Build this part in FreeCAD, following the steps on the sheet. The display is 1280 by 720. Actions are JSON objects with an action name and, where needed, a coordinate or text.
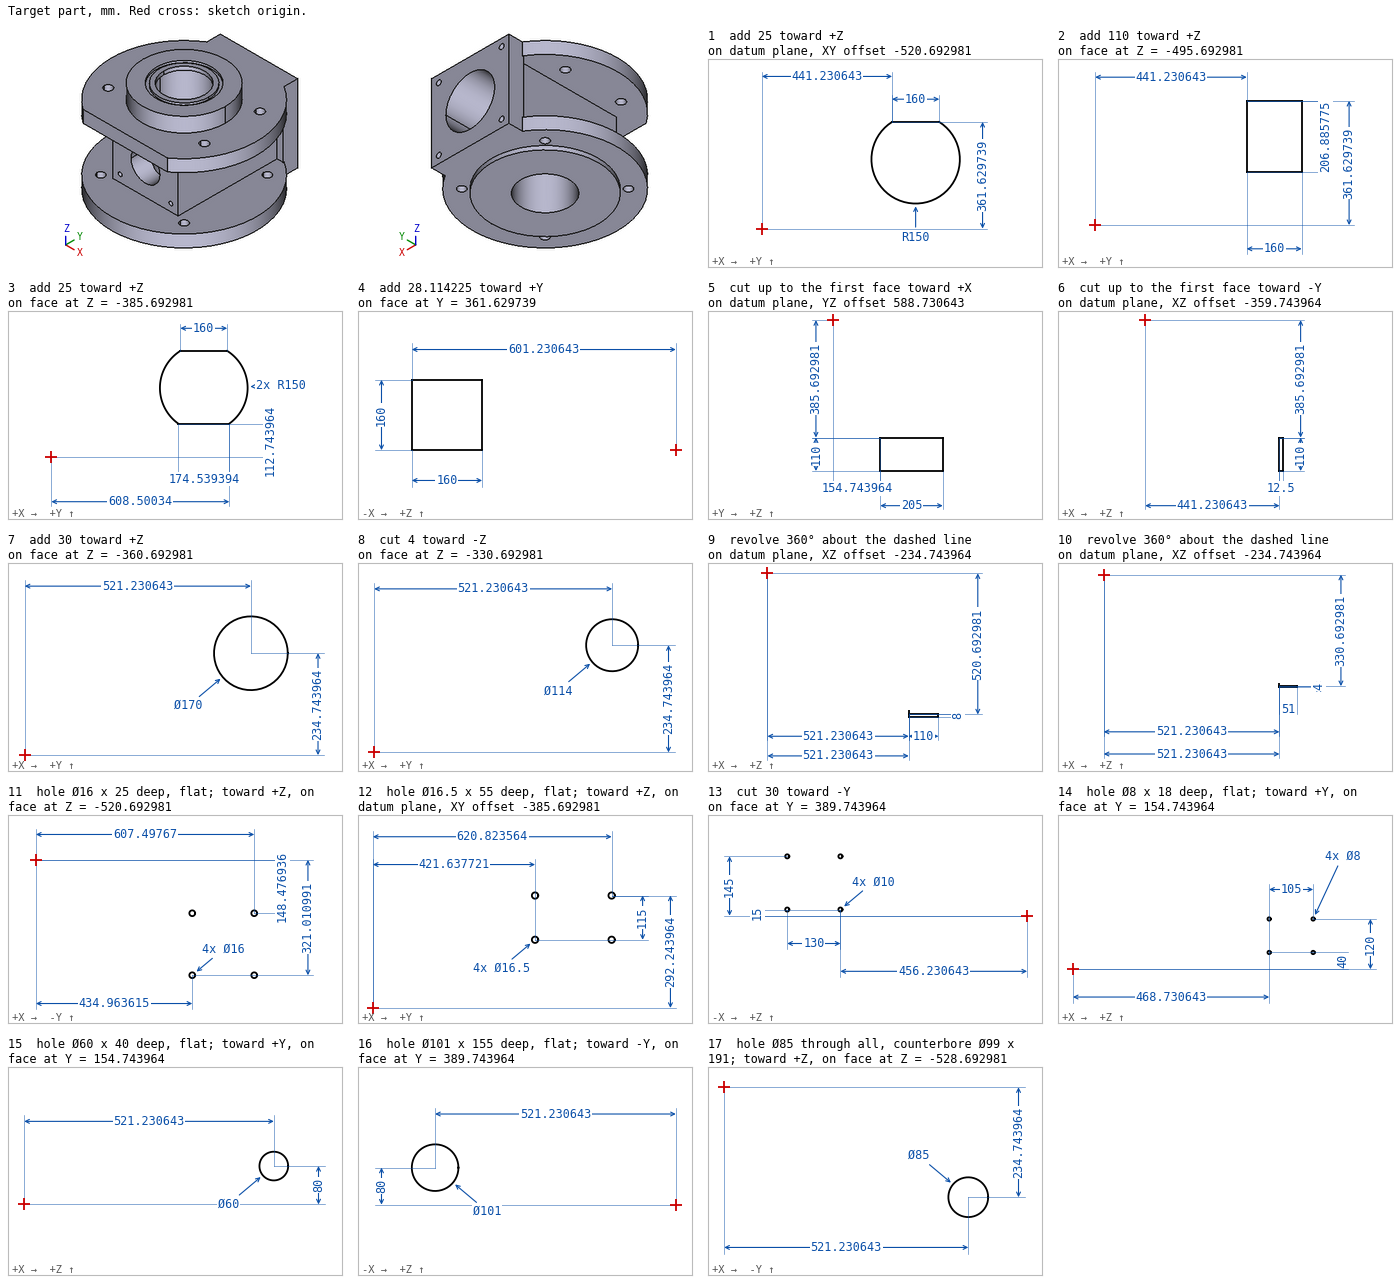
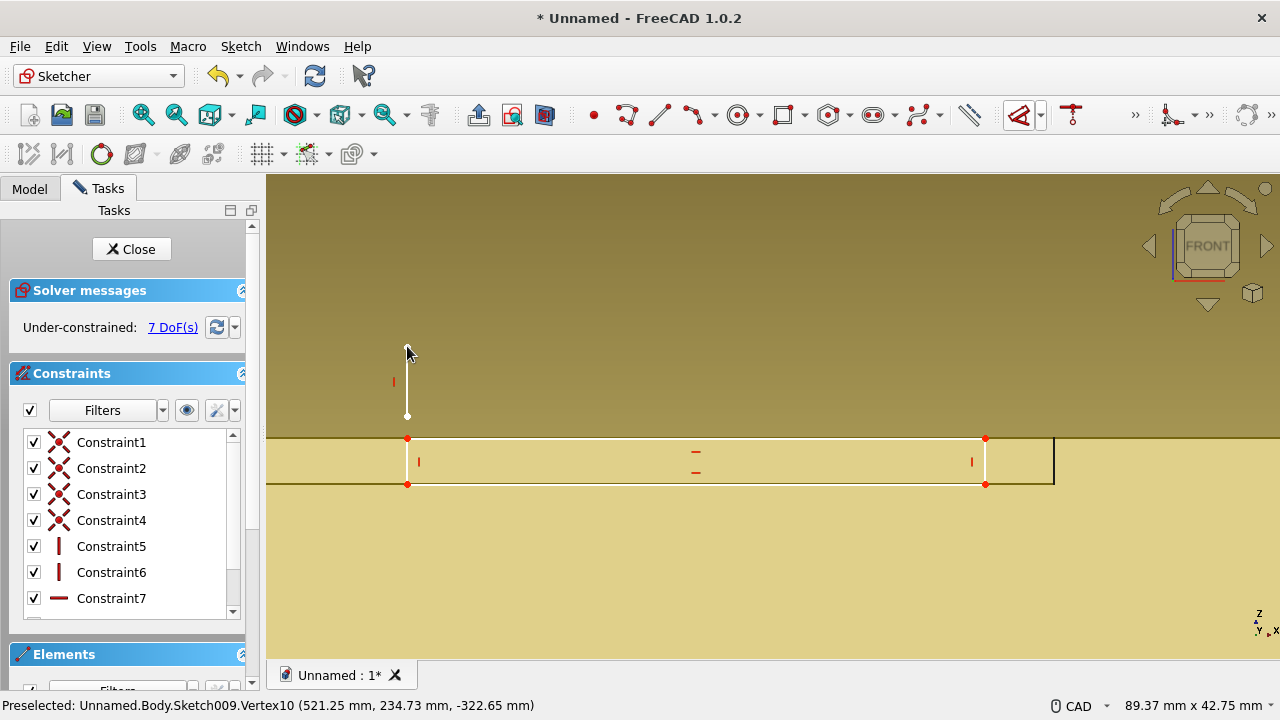
{"action": "left_click", "coordinate": [407, 395]}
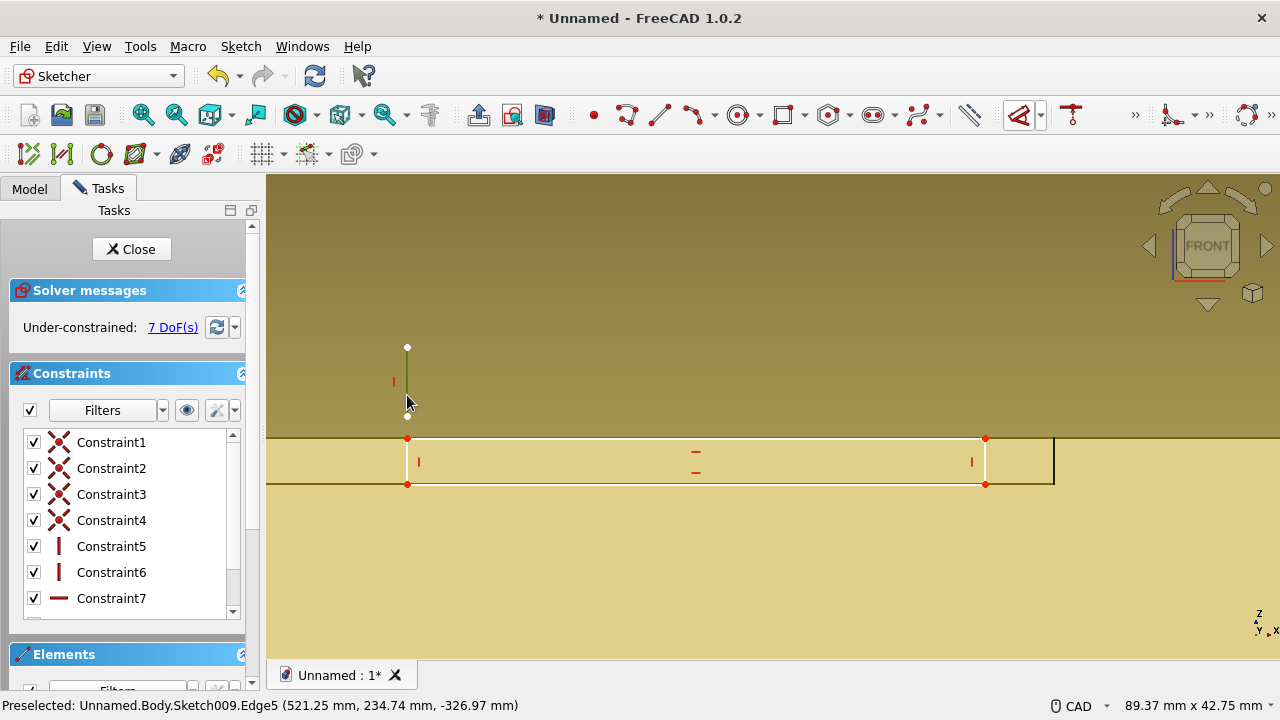
{"action": "left_click", "coordinate": [970, 116]}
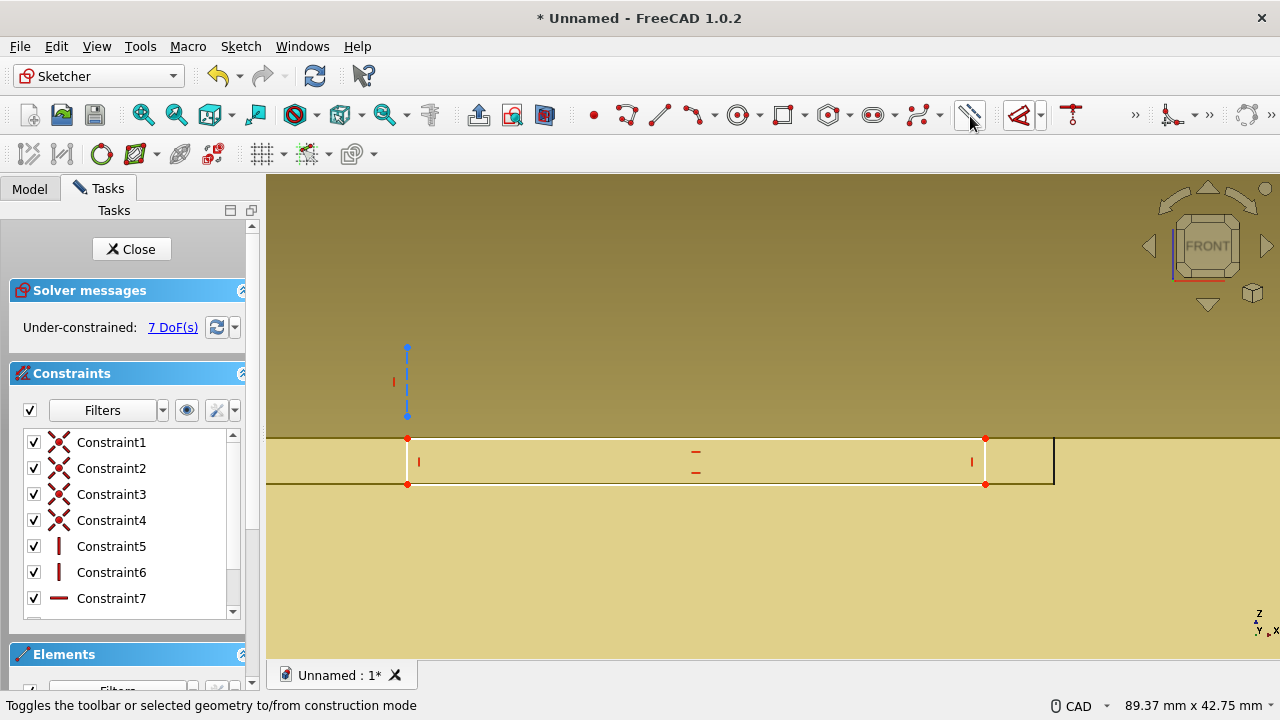
{"action": "left_click", "coordinate": [407, 453]}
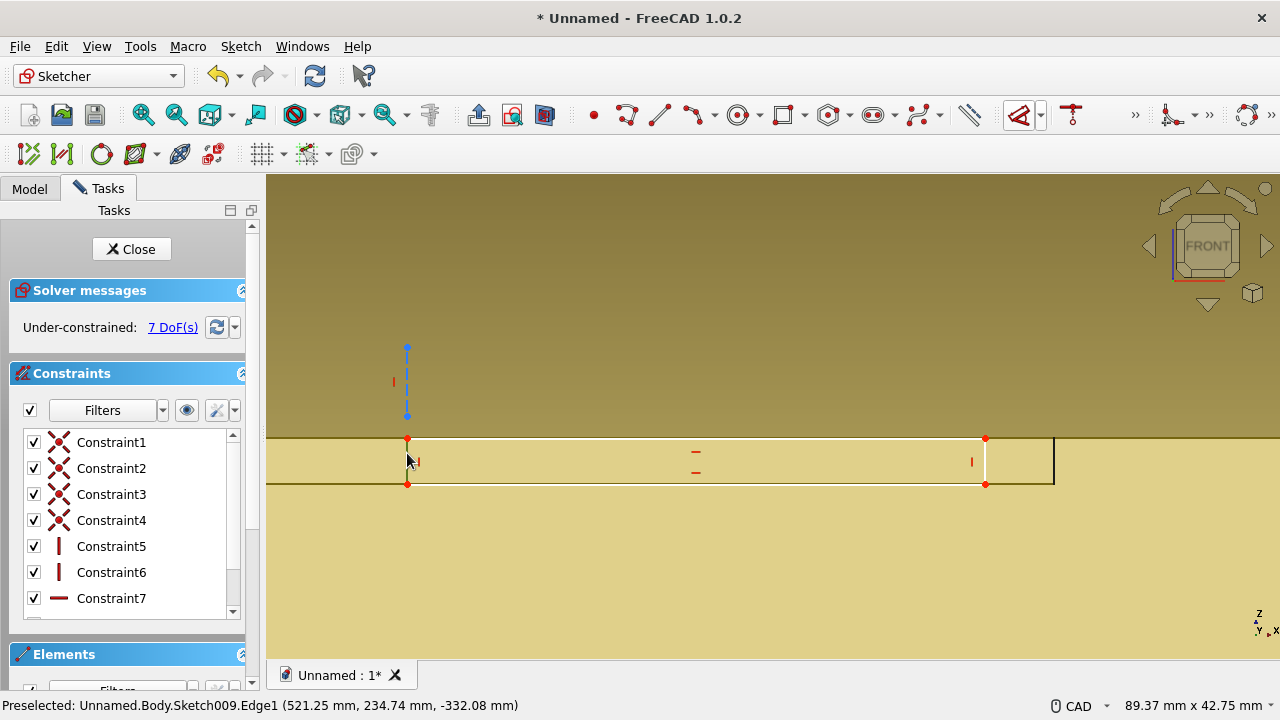
{"action": "key", "text": "i"}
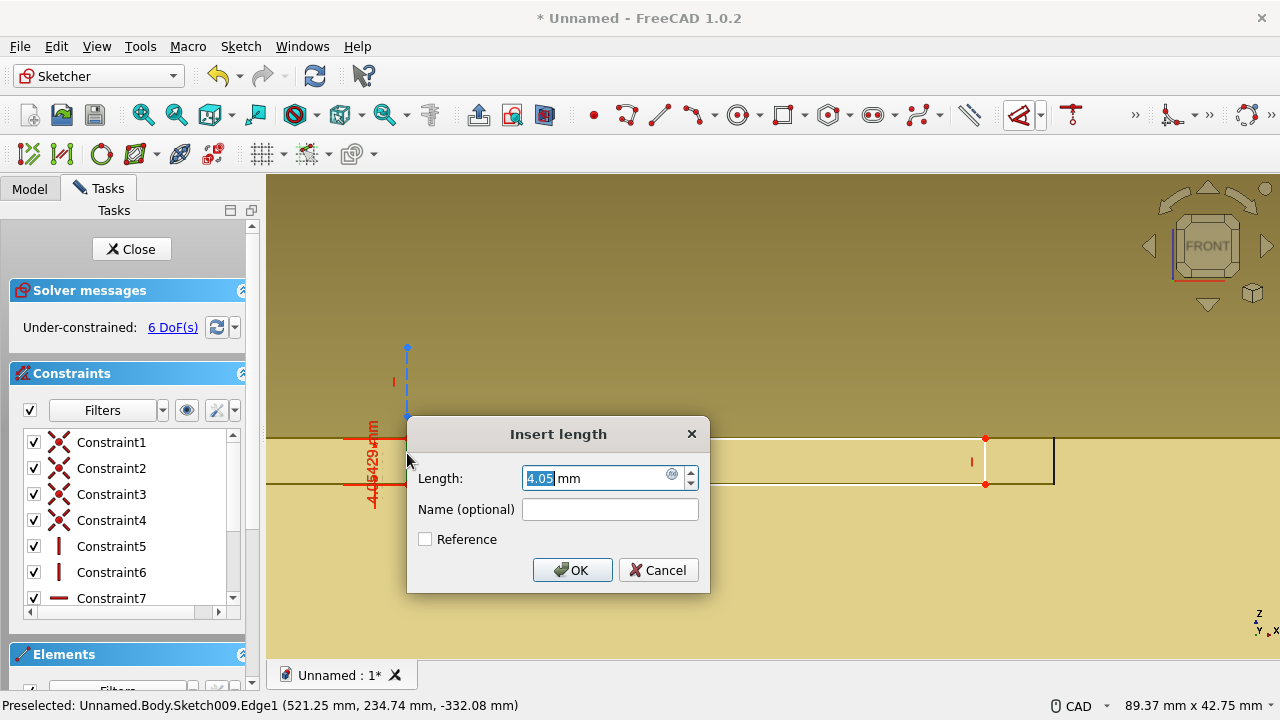
{"action": "type", "text": "4"}
{"action": "key", "text": "Return"}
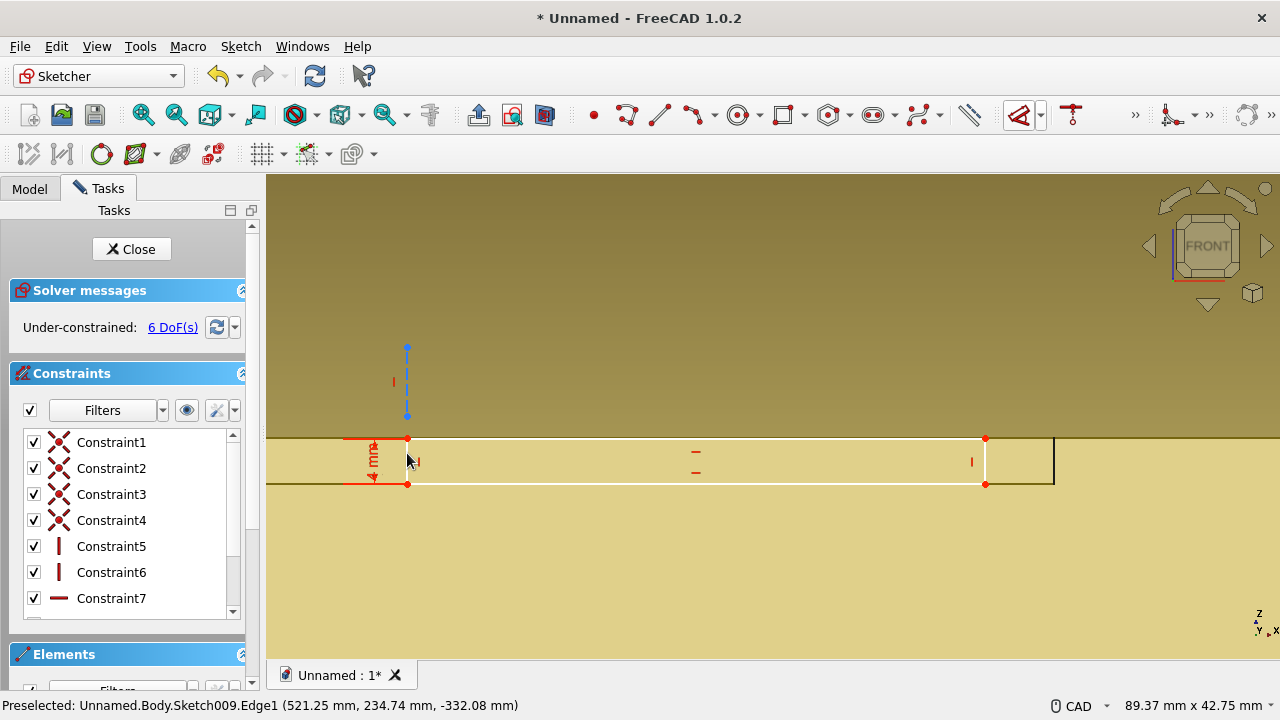
{"action": "left_click", "coordinate": [580, 484]}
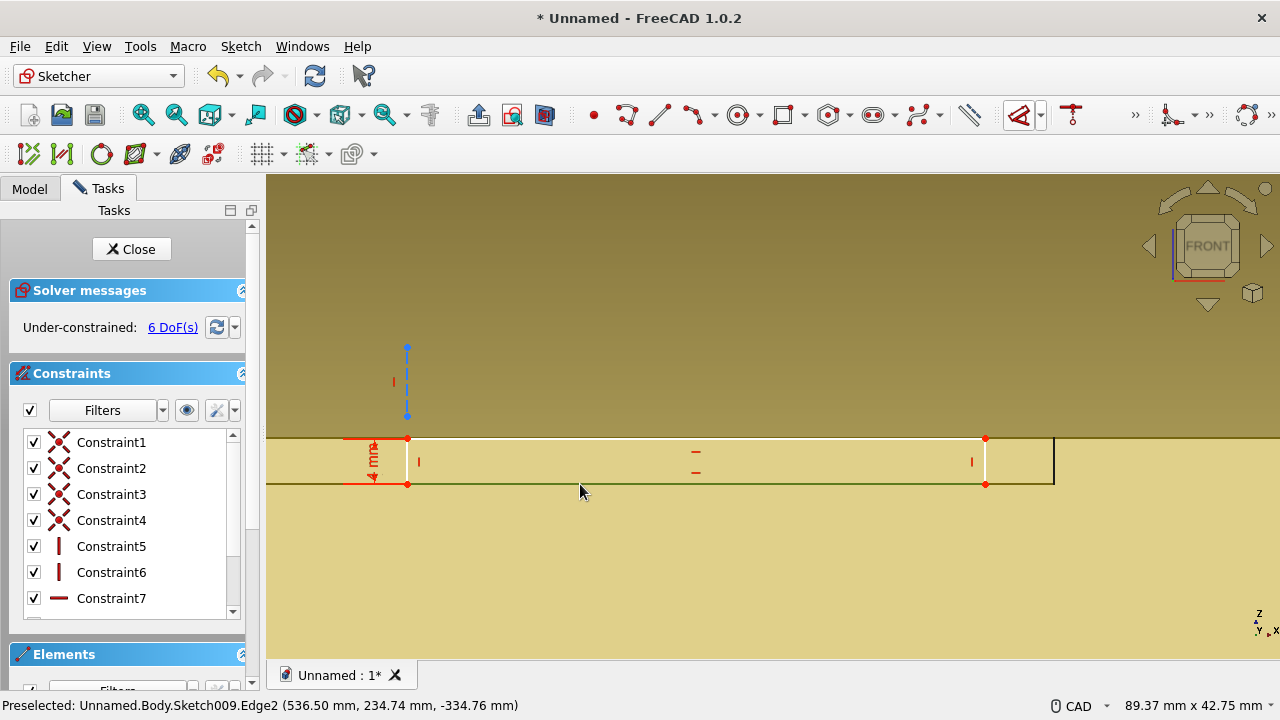
{"action": "key", "text": "l"}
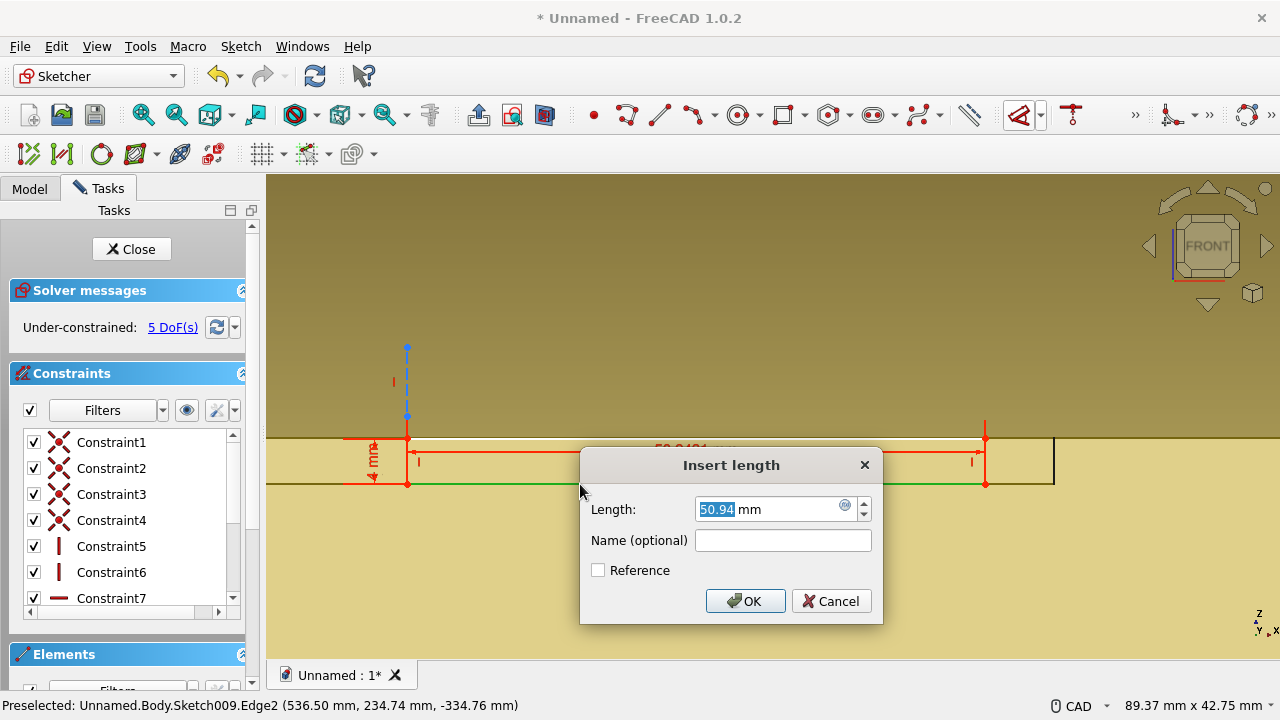
{"action": "type", "text": "51"}
{"action": "key", "text": "Return"}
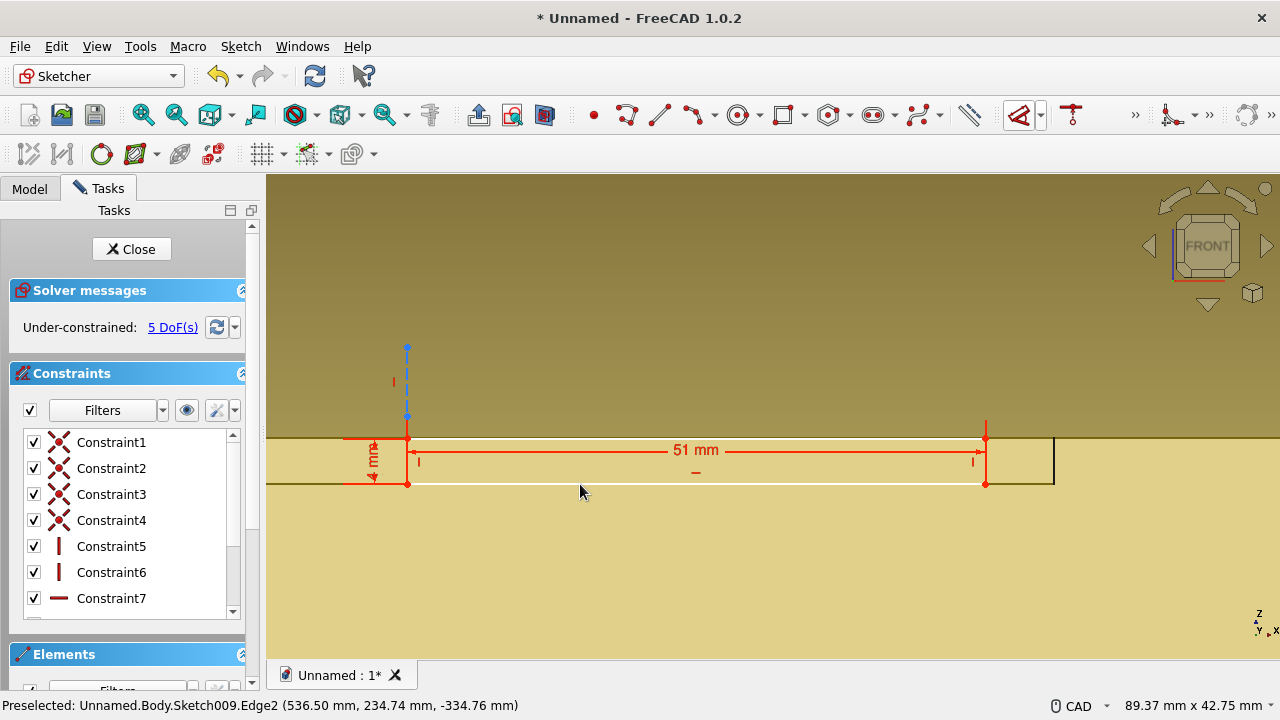
{"action": "left_click", "coordinate": [407, 439]}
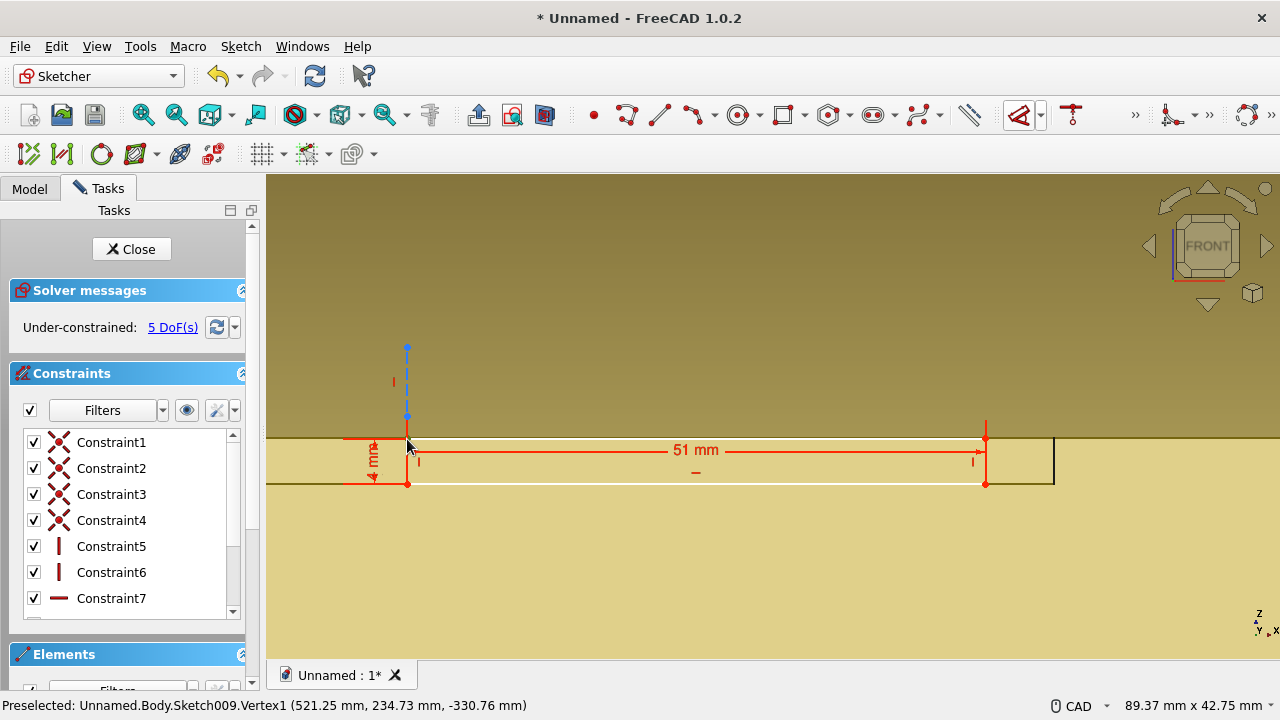
{"action": "key", "text": "l"}